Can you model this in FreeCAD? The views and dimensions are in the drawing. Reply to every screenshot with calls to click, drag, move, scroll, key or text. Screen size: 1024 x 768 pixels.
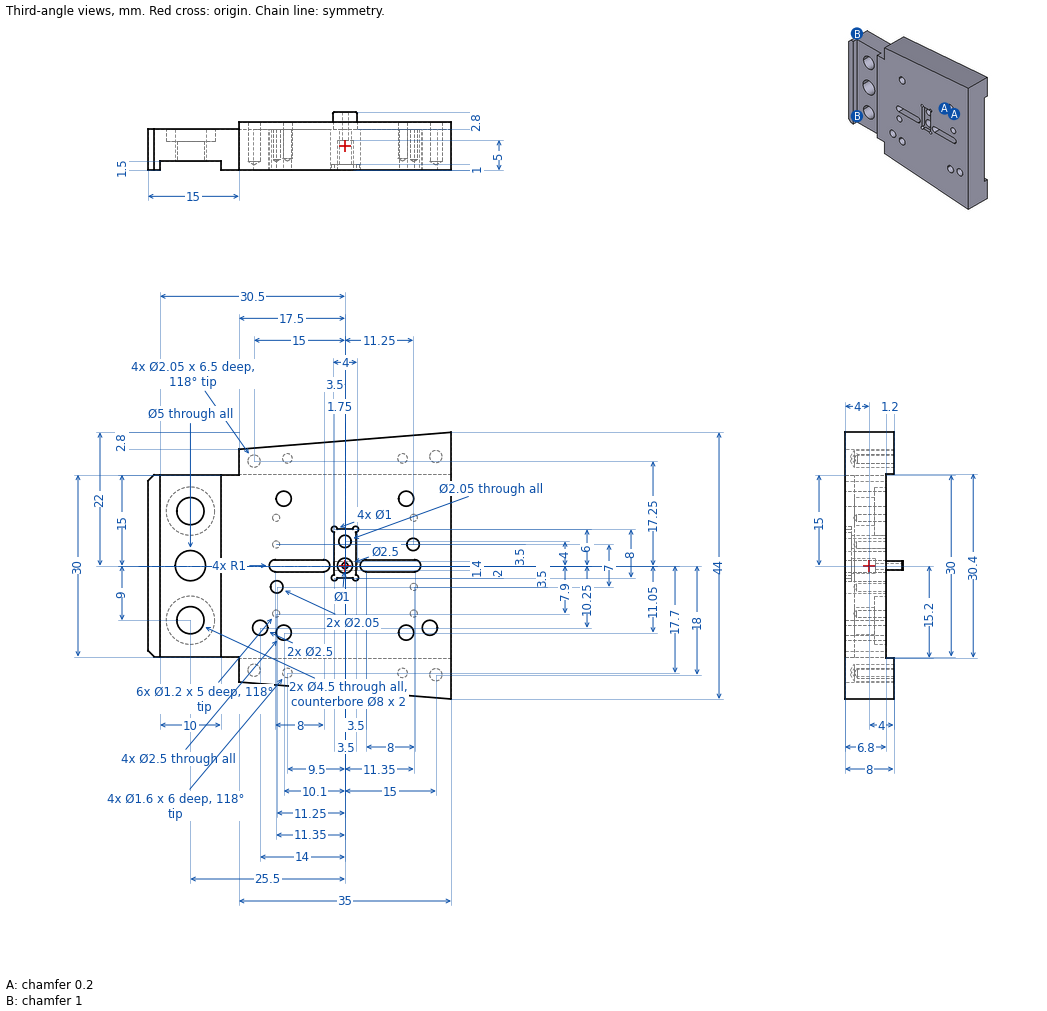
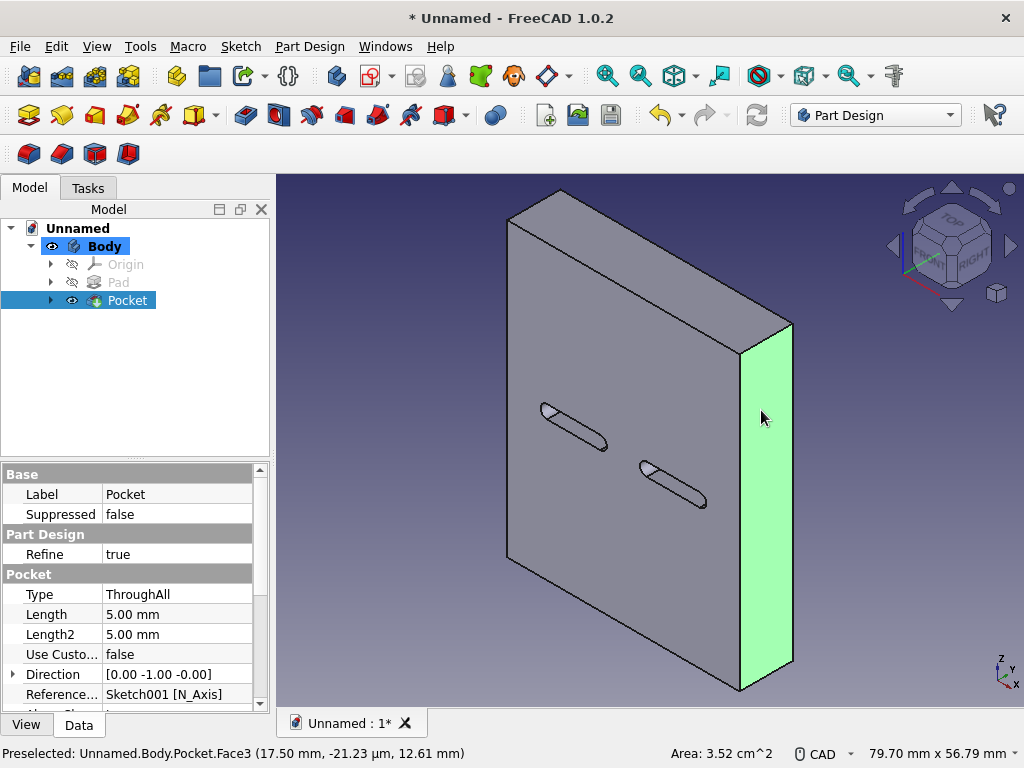
click(370, 76)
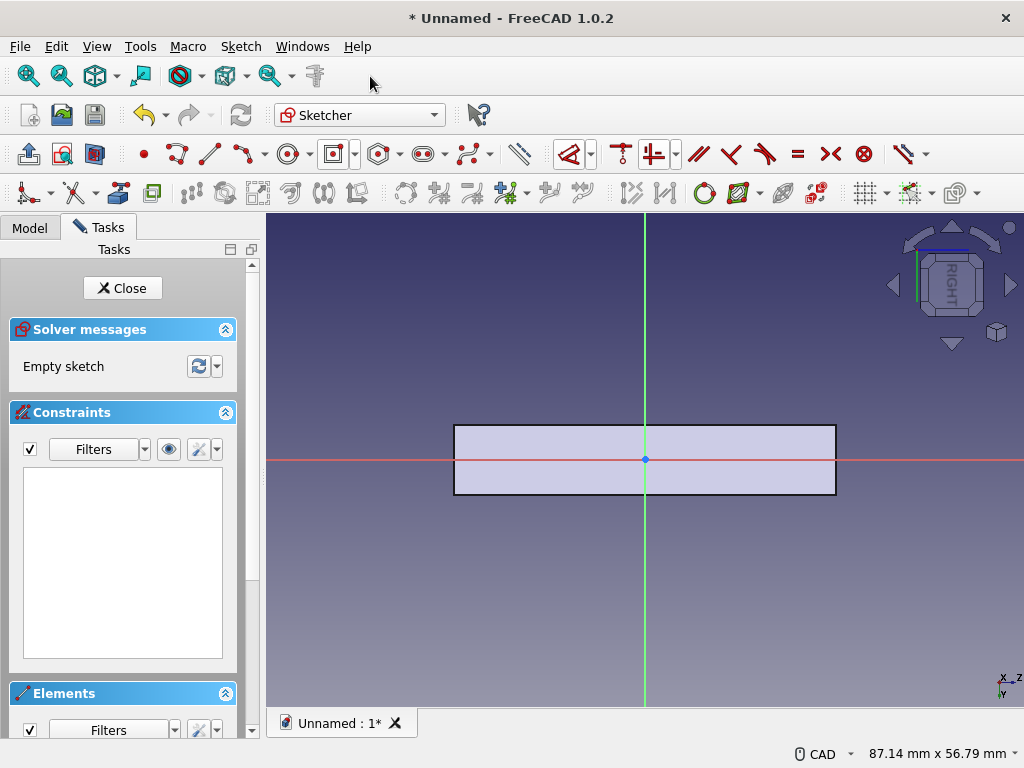
scroll(784, 513, up, 2)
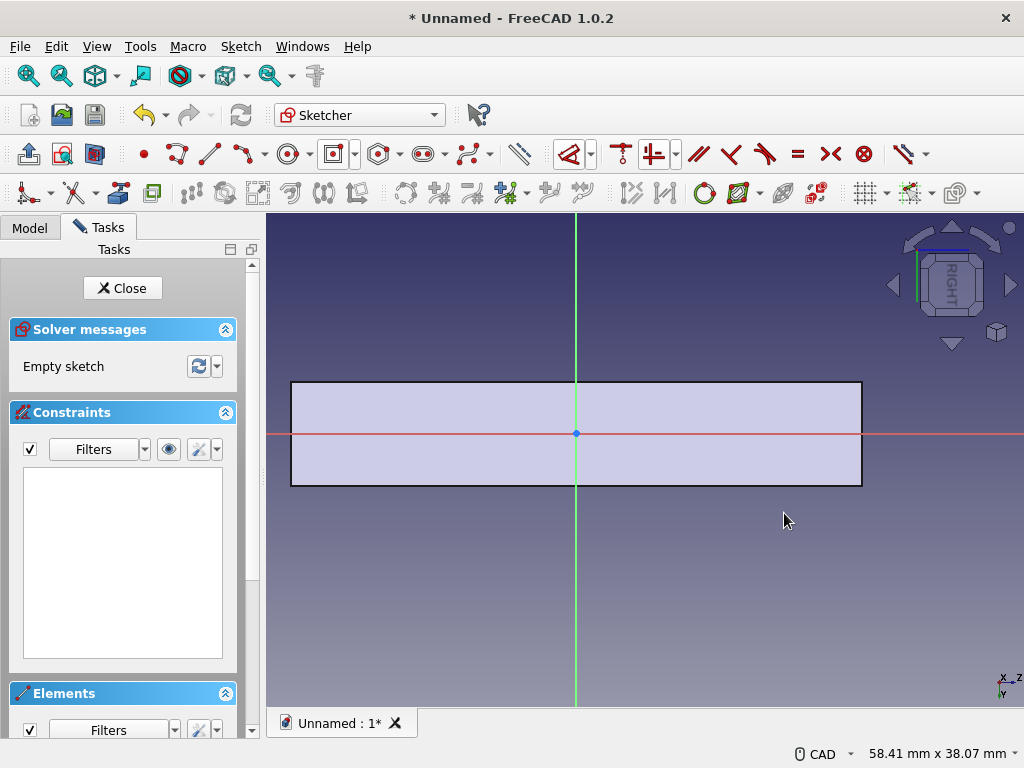
click(354, 154)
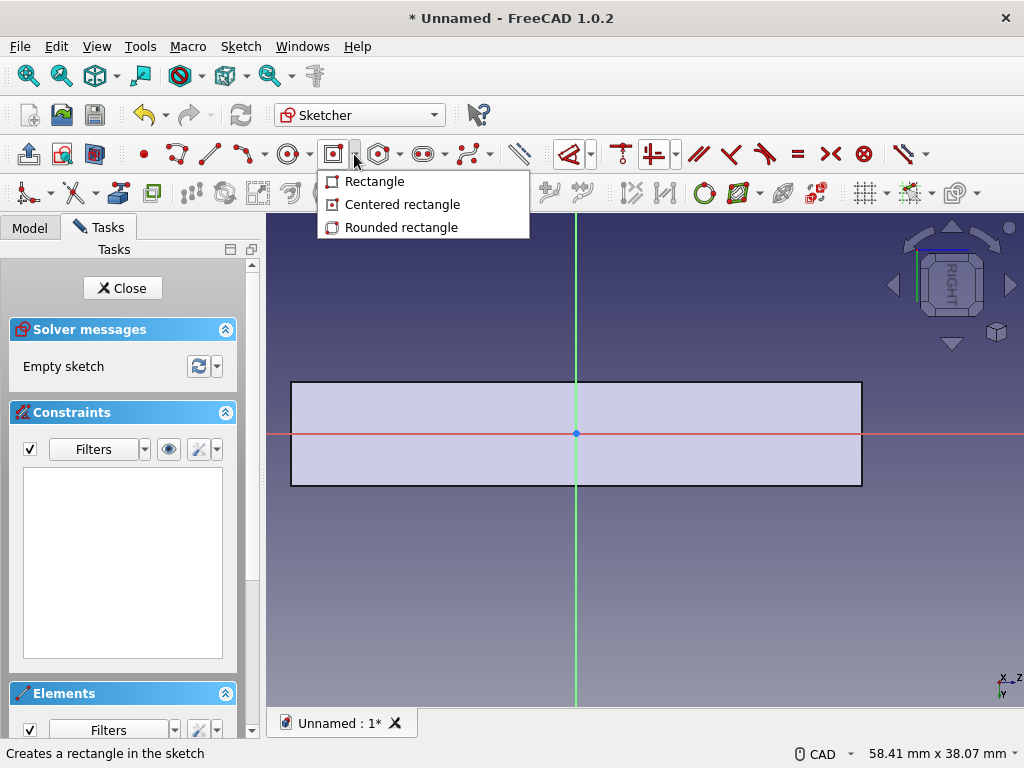
click(424, 182)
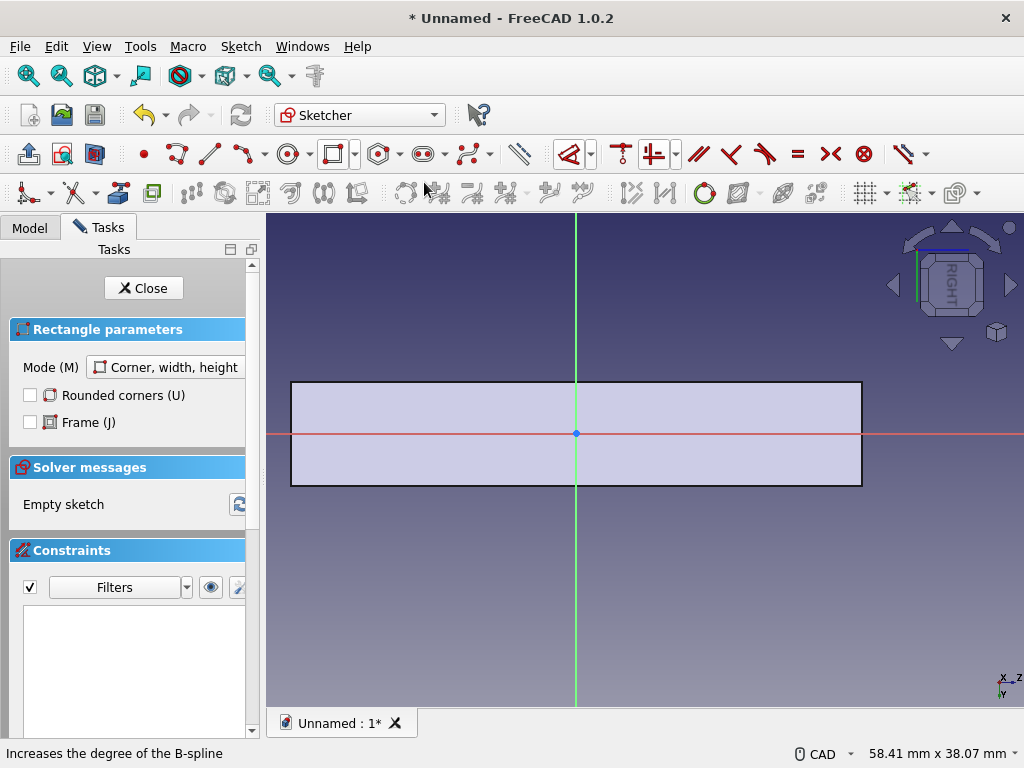
click(379, 470)
move(774, 486)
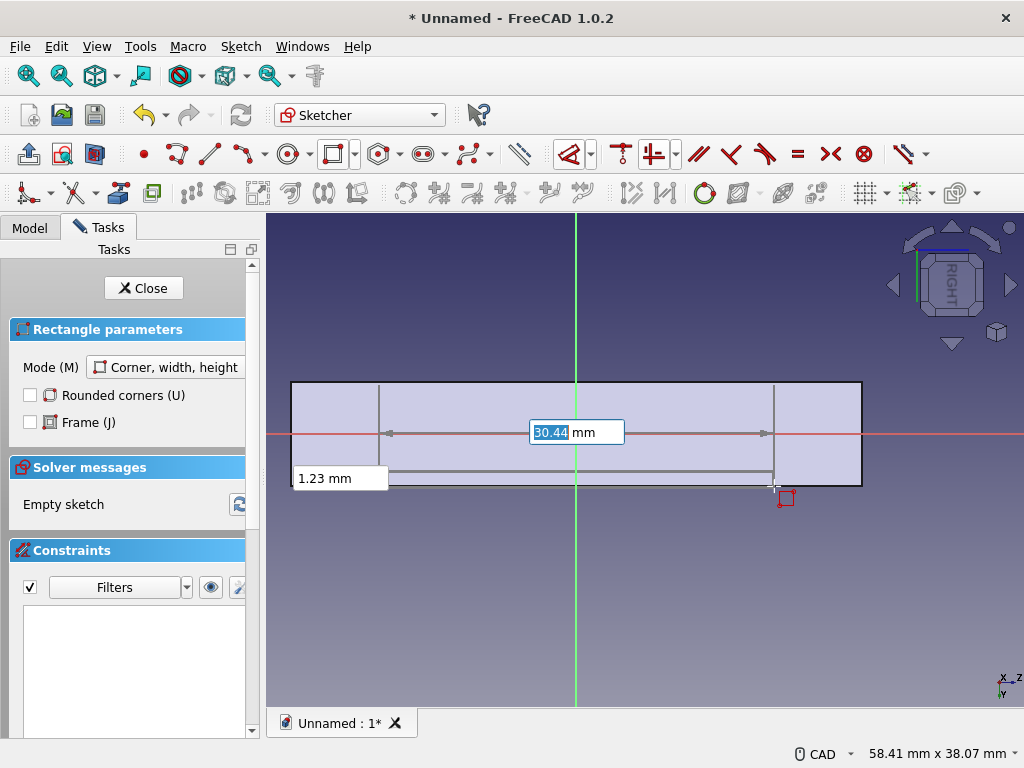
text(30.4)
key(Tab)
text(1.2)
key(Return)
key(Escape)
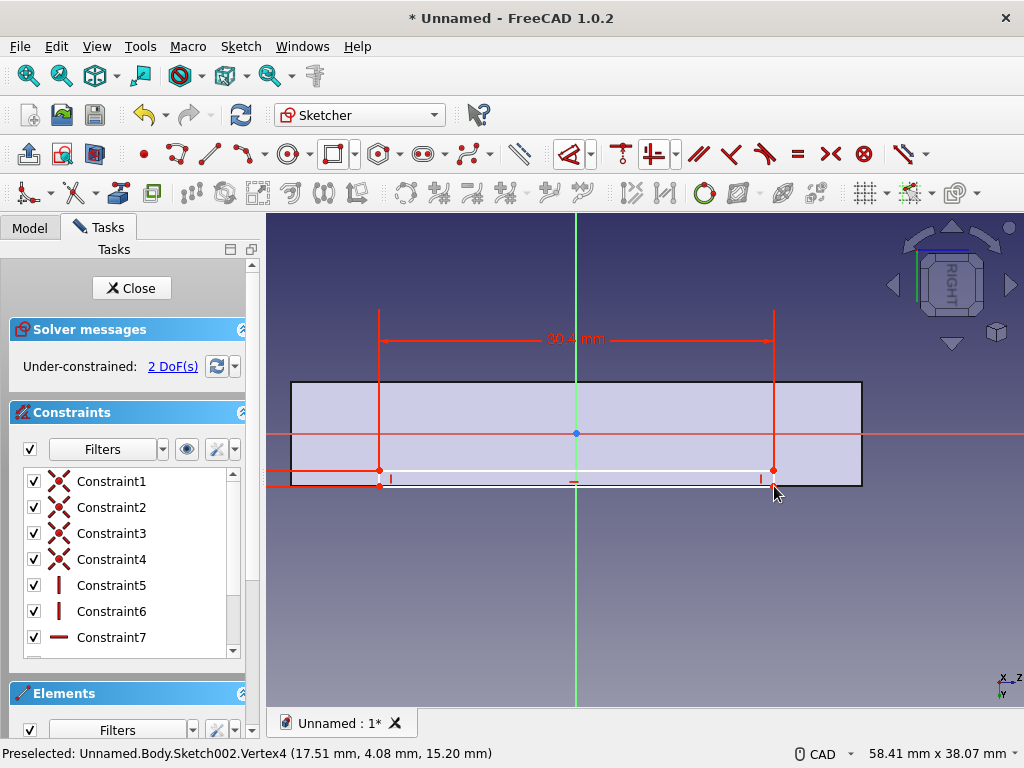
click(379, 487)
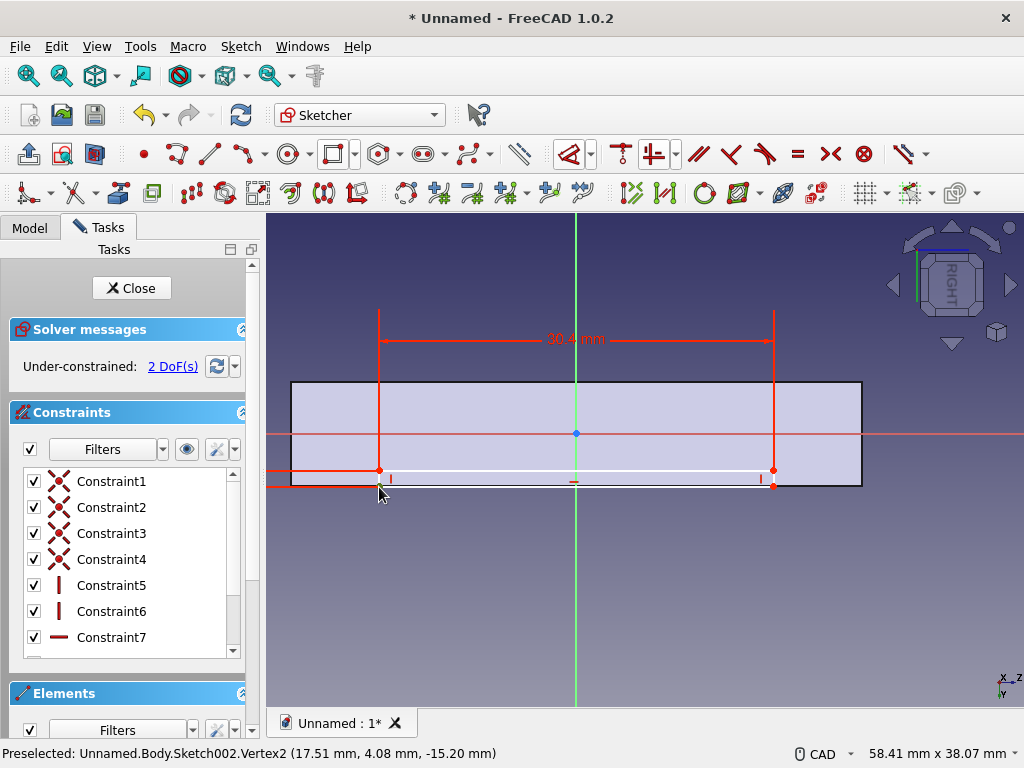
click(590, 154)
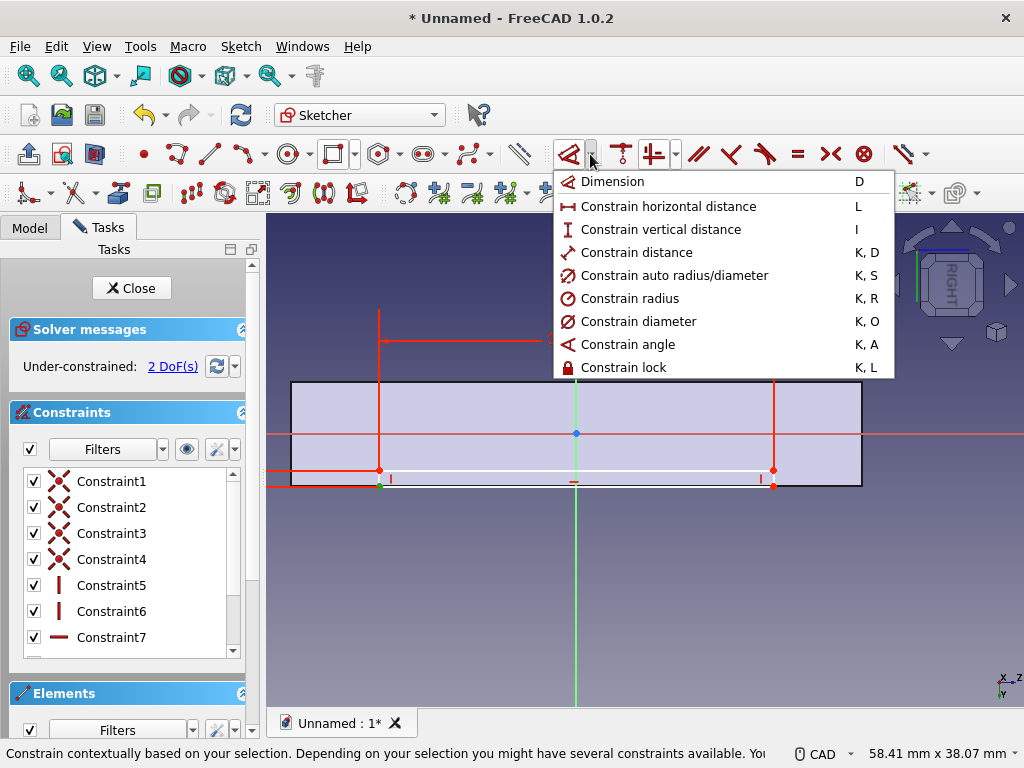
click(724, 230)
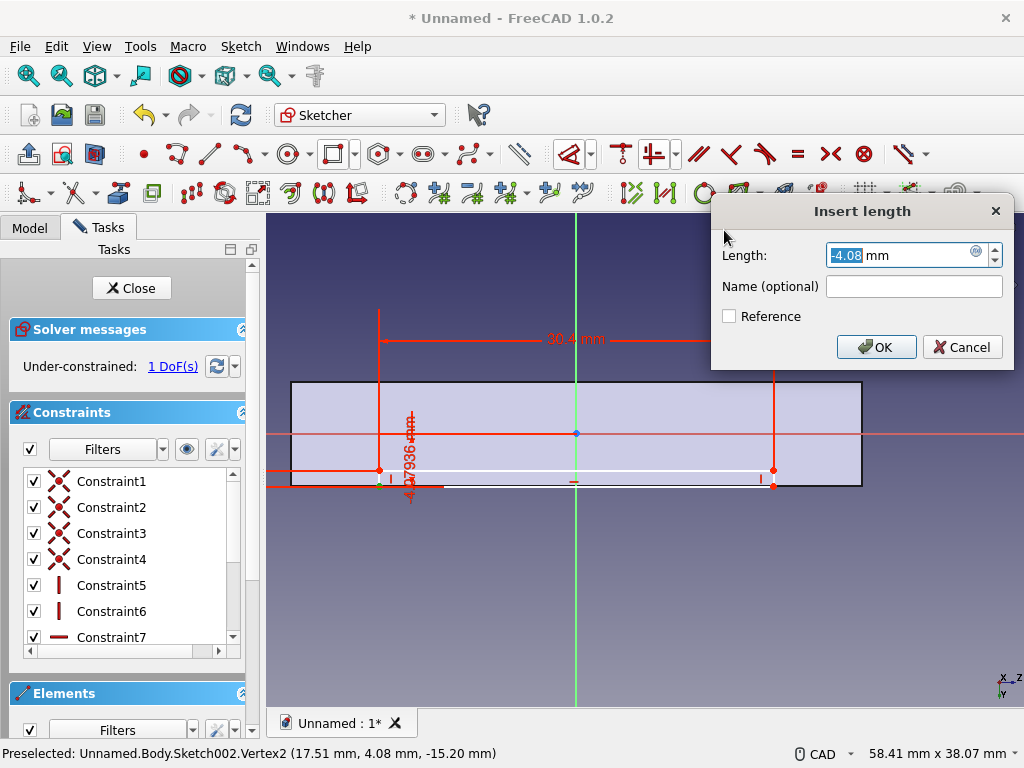
text(-4)
key(Return)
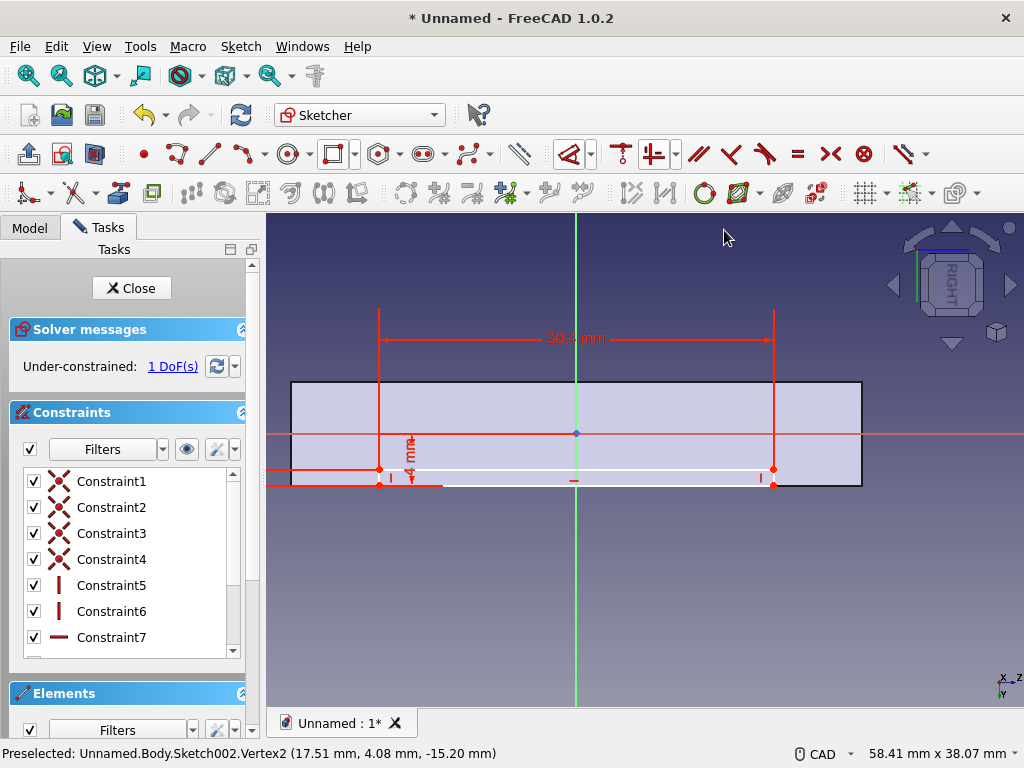
click(379, 470)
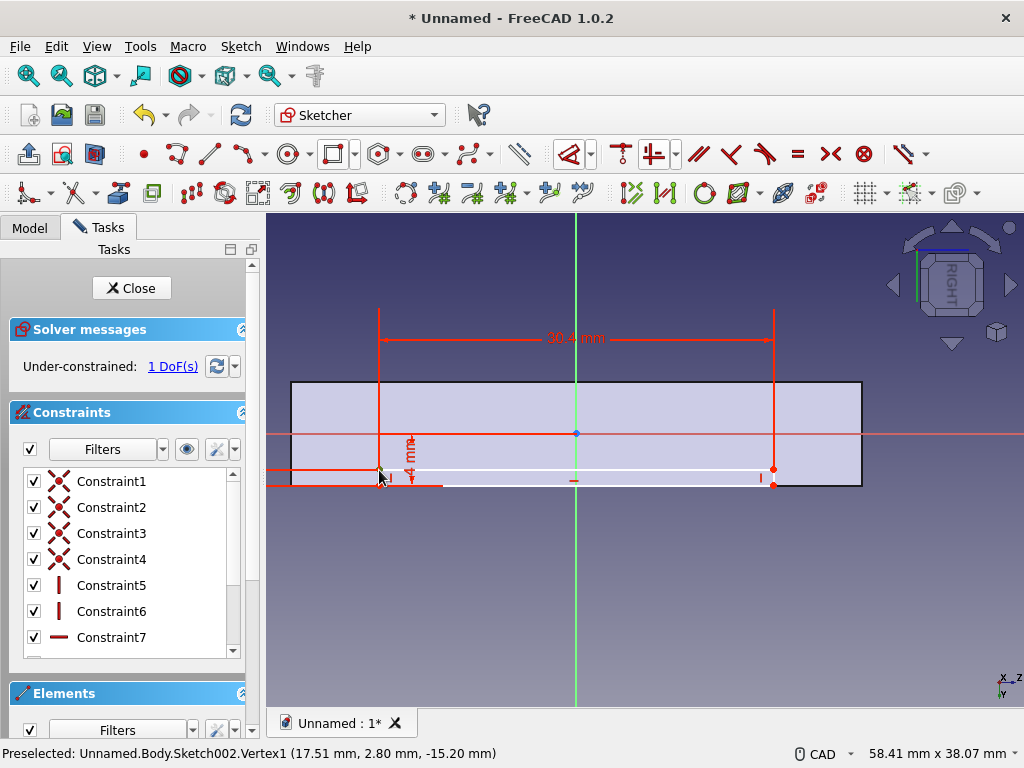
key(l)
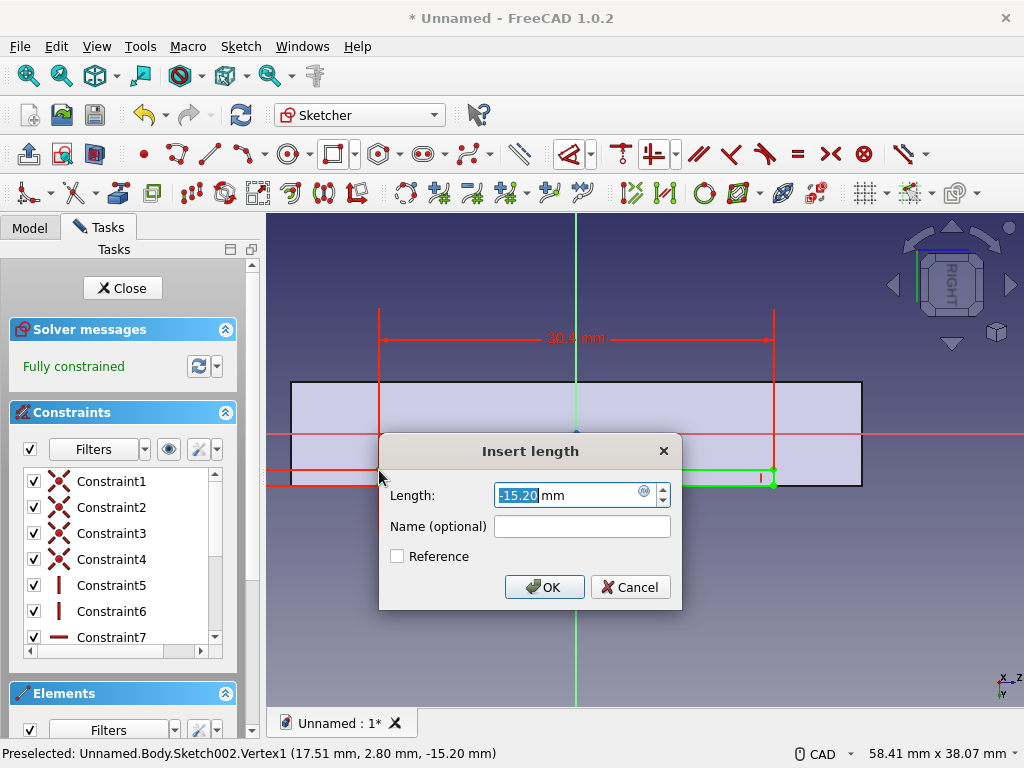
text(-15.2)
key(Return)